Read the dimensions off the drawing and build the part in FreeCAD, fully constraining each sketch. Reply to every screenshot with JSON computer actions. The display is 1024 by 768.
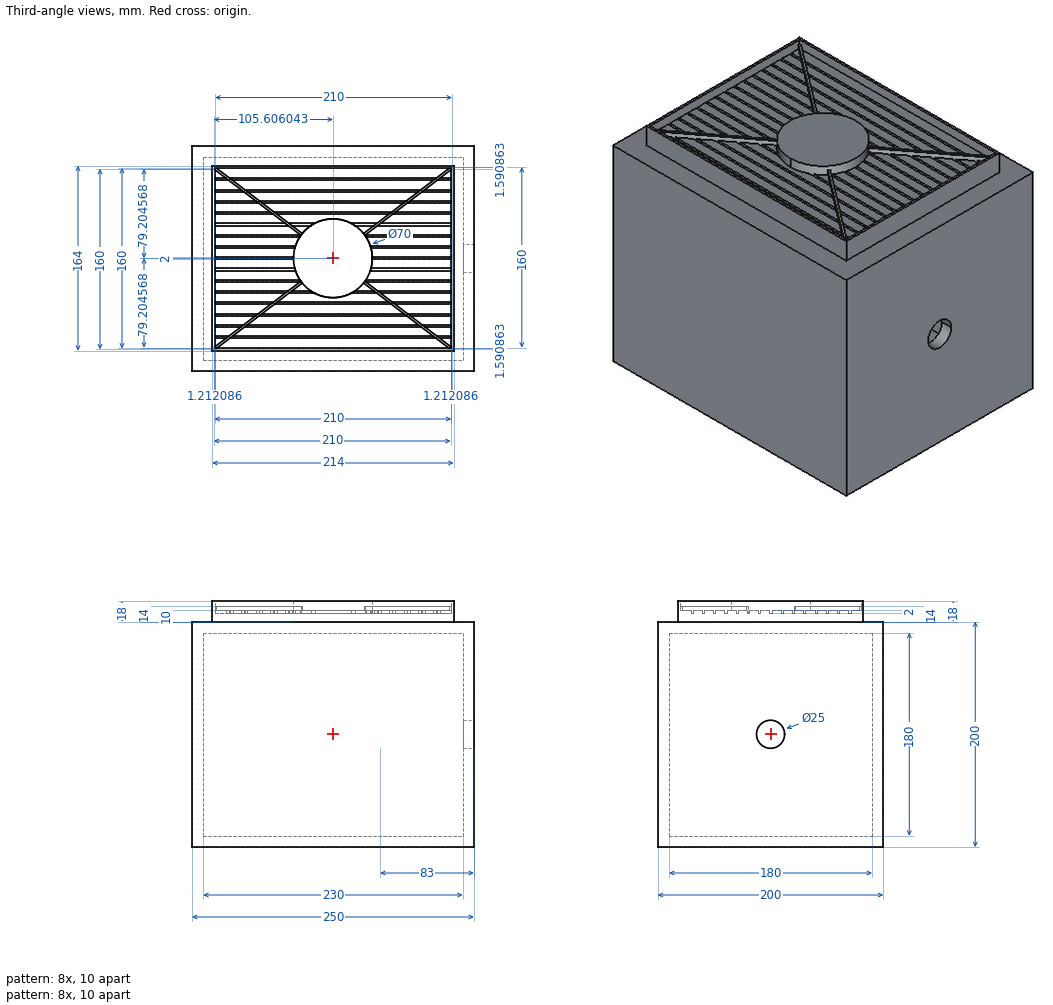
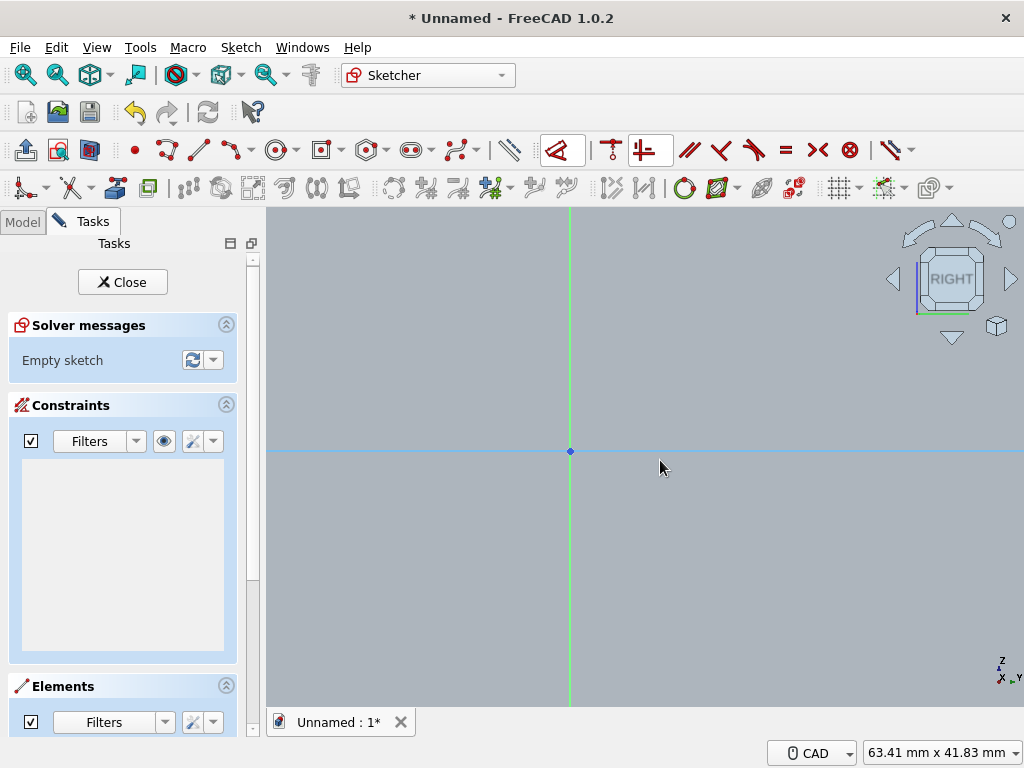
{"action": "left_click", "coordinate": [276, 150]}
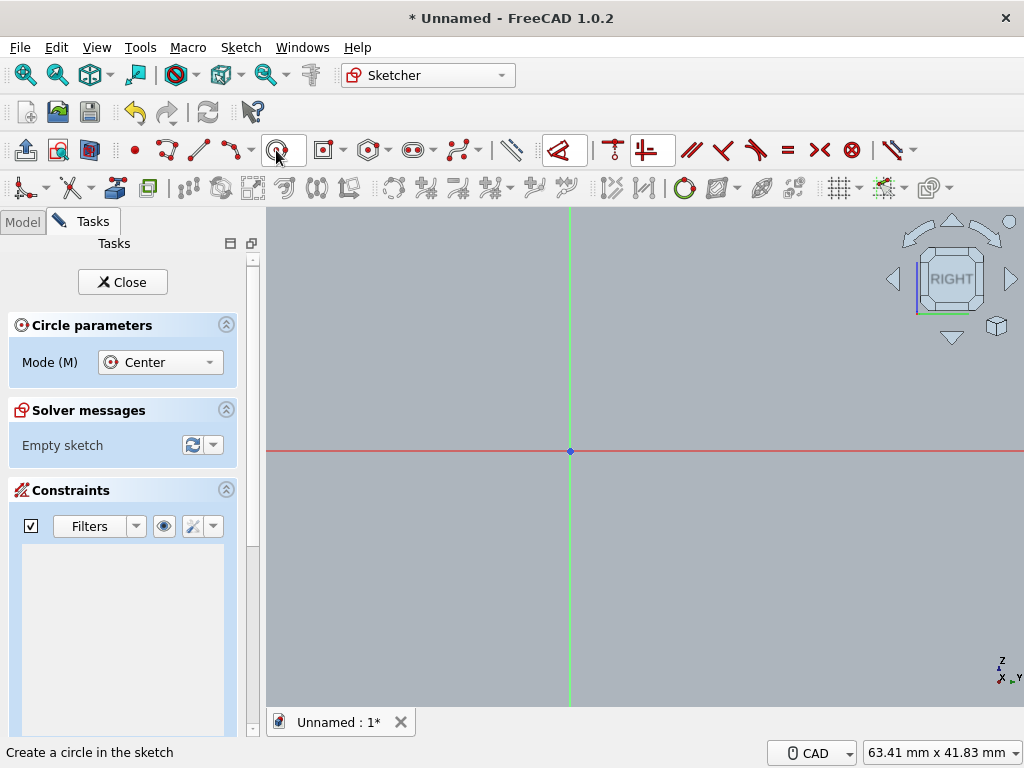
{"action": "left_click", "coordinate": [570, 451]}
{"action": "left_click", "coordinate": [676, 345]}
{"action": "key", "text": "Escape"}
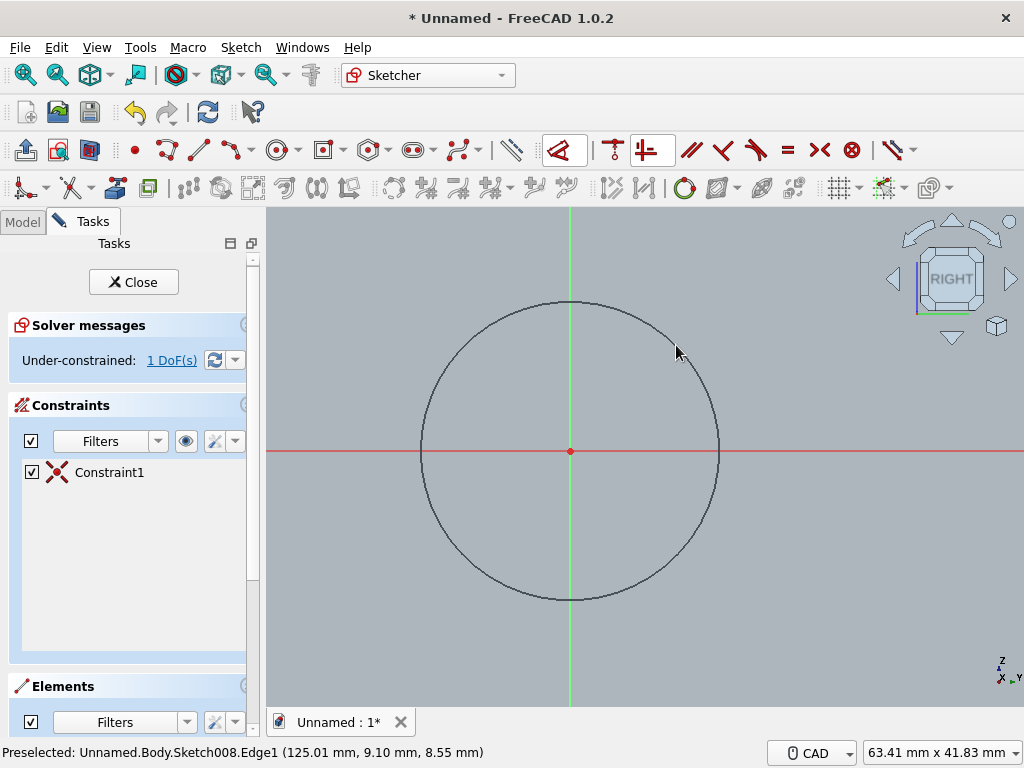
{"action": "left_click", "coordinate": [675, 345]}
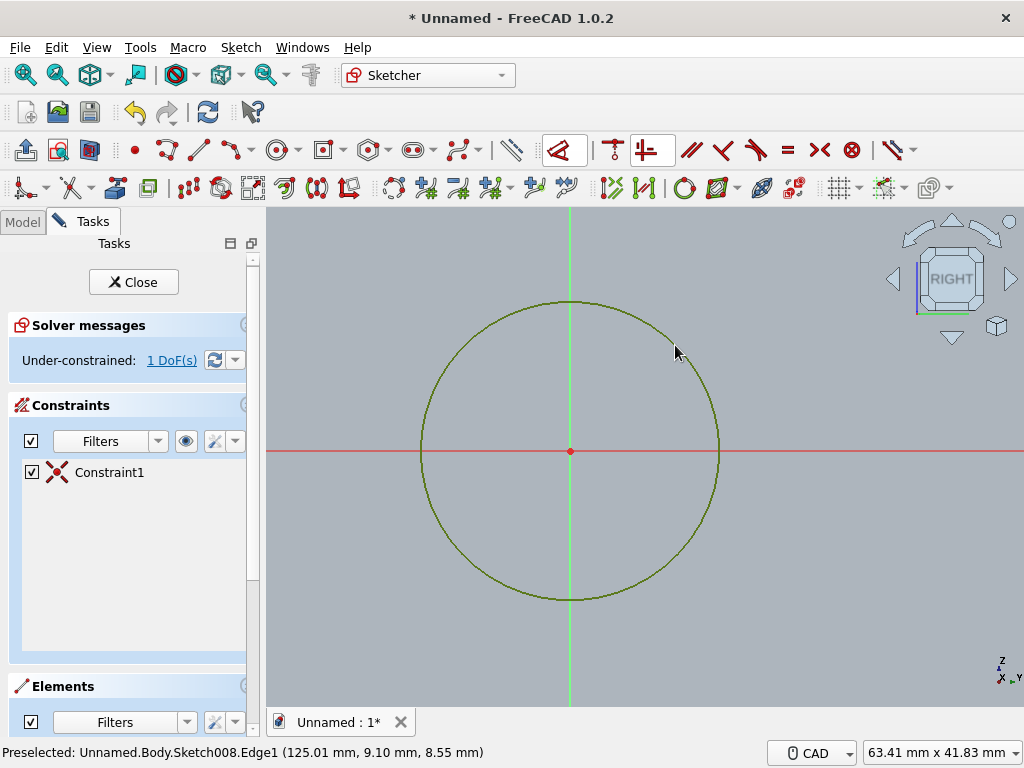
{"action": "left_click", "coordinate": [582, 150]}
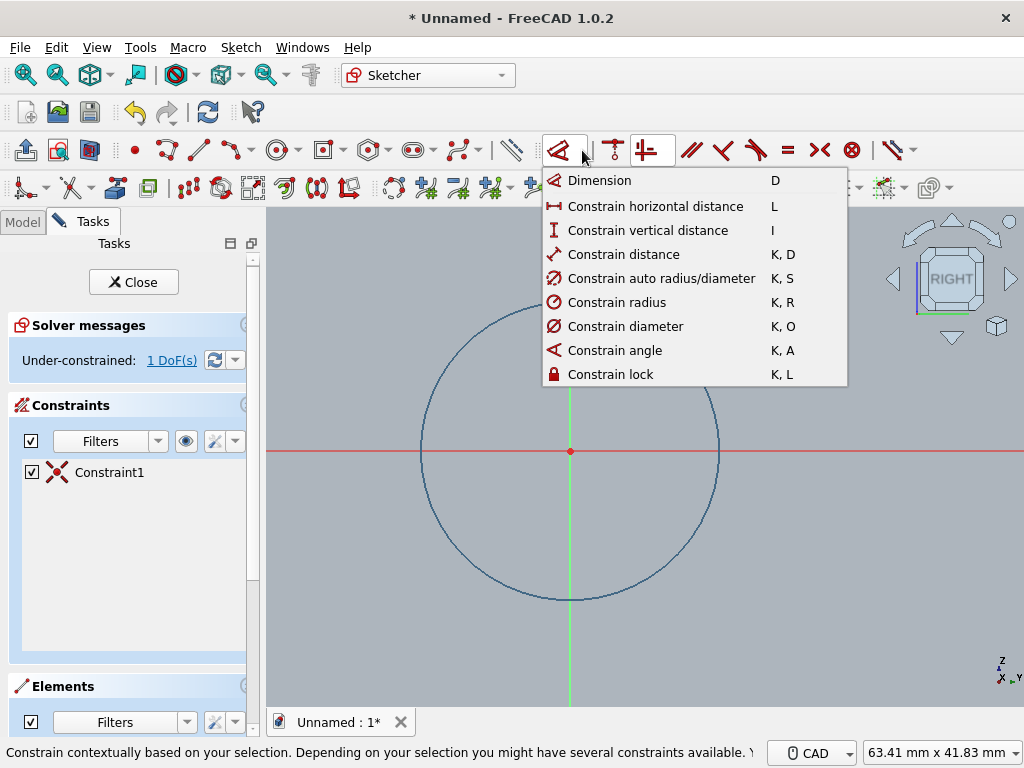
{"action": "left_click", "coordinate": [695, 326]}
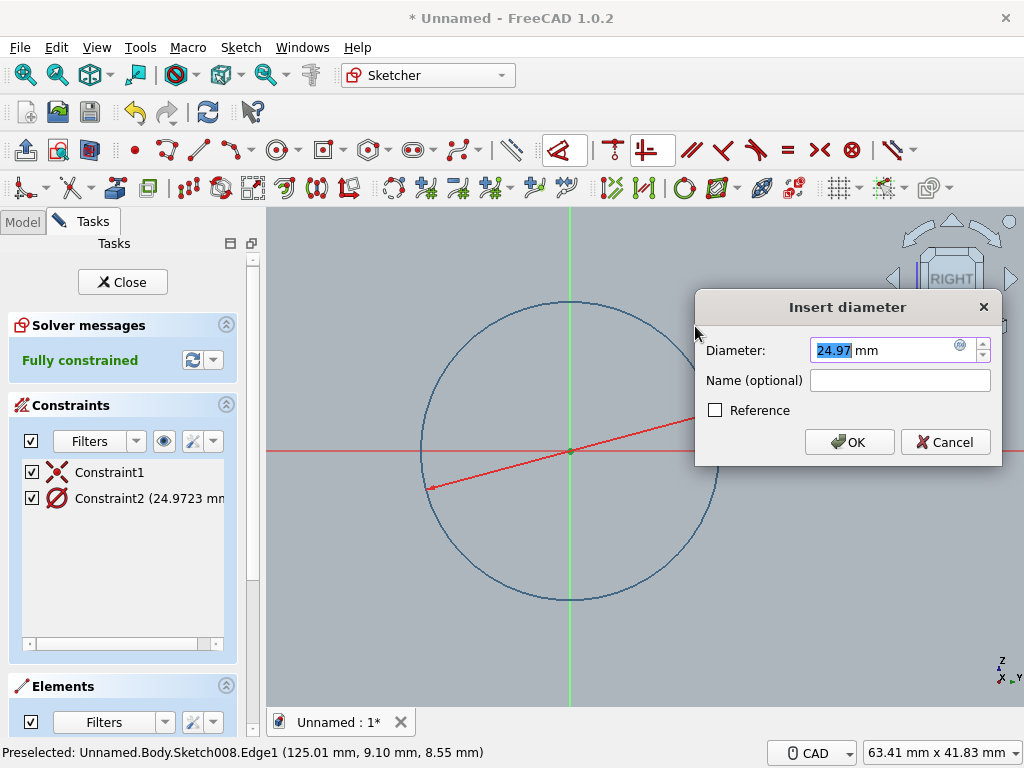
{"action": "type", "text": "25"}
{"action": "key", "text": "Return"}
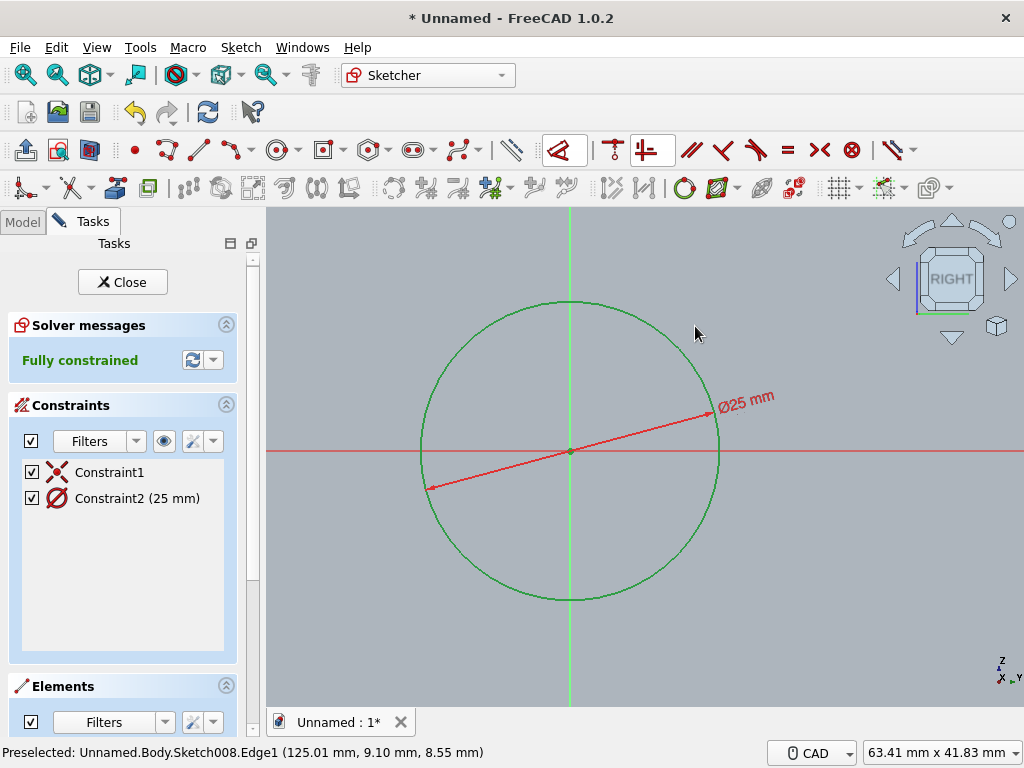
{"action": "left_click", "coordinate": [123, 282]}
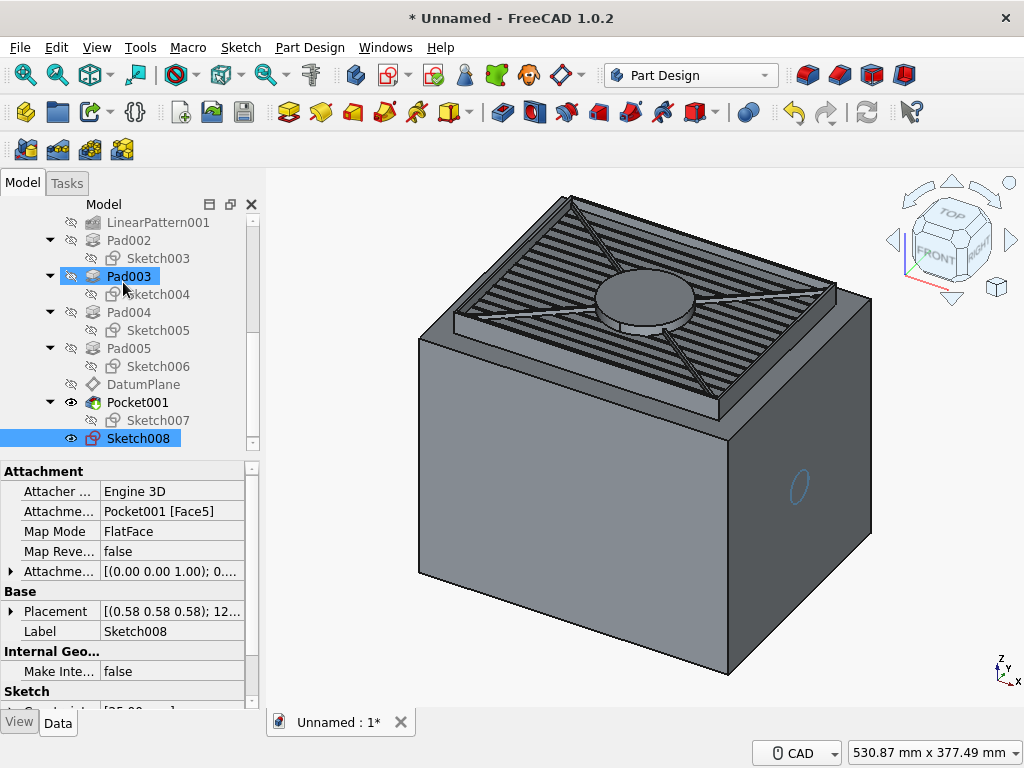
{"action": "left_click", "coordinate": [504, 112]}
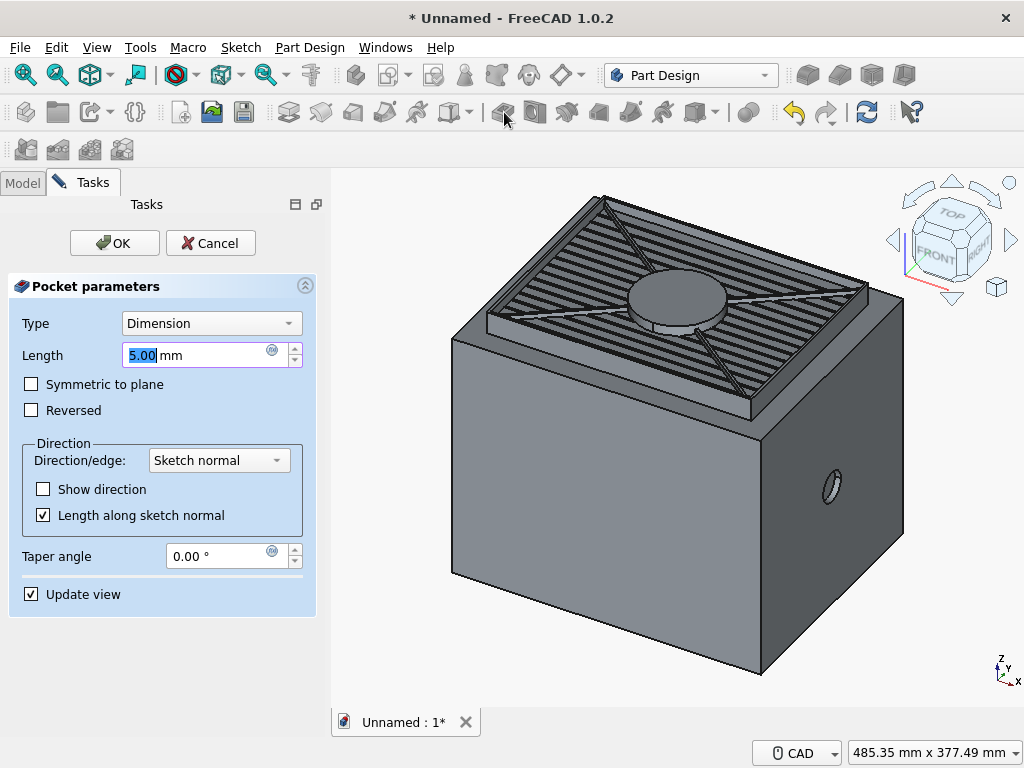
{"action": "type", "text": "83"}
{"action": "key", "text": "Tab"}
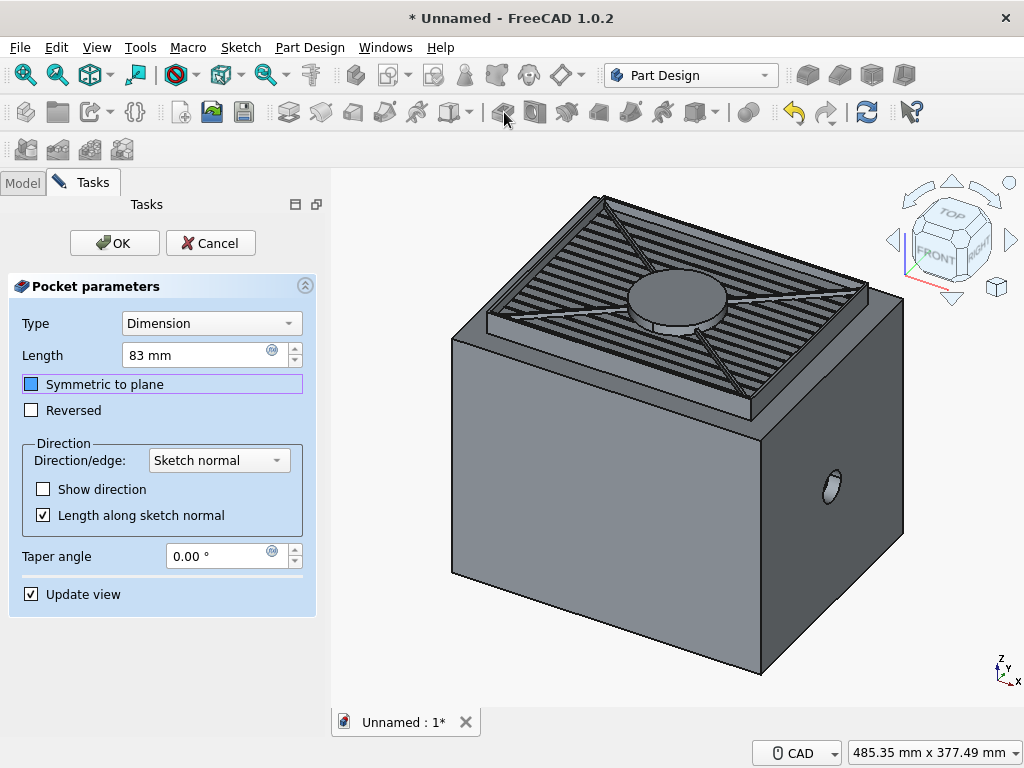
{"action": "left_click", "coordinate": [115, 243]}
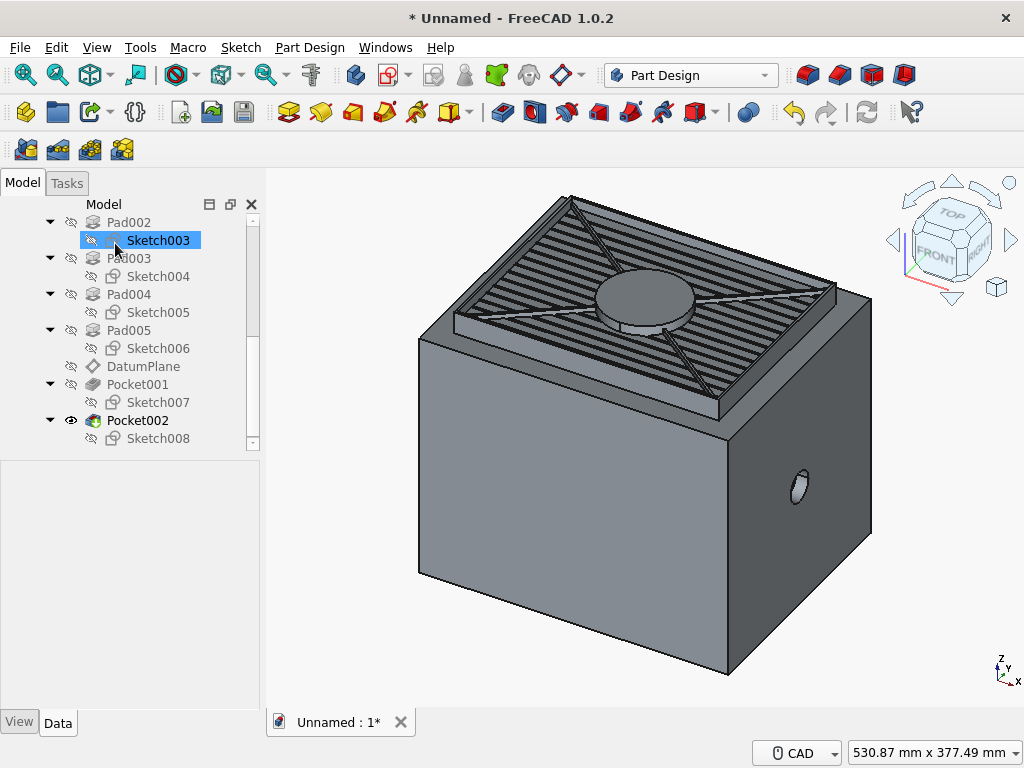
{"action": "key", "text": "0"}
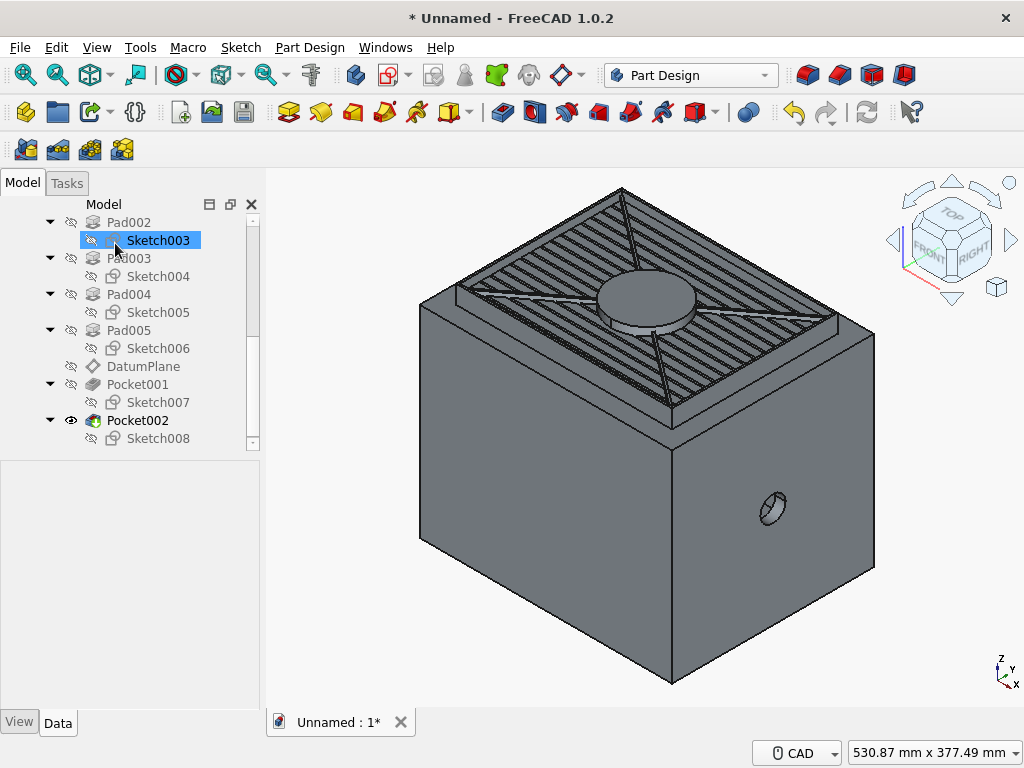
{"action": "left_click", "coordinate": [26, 76]}